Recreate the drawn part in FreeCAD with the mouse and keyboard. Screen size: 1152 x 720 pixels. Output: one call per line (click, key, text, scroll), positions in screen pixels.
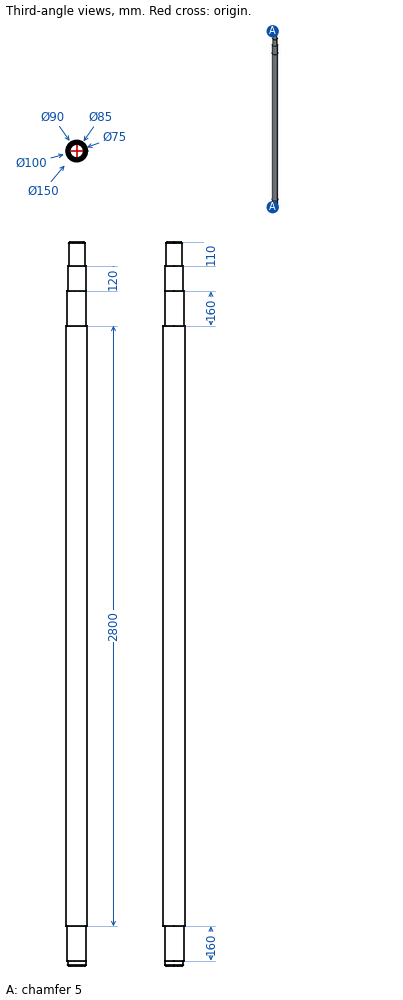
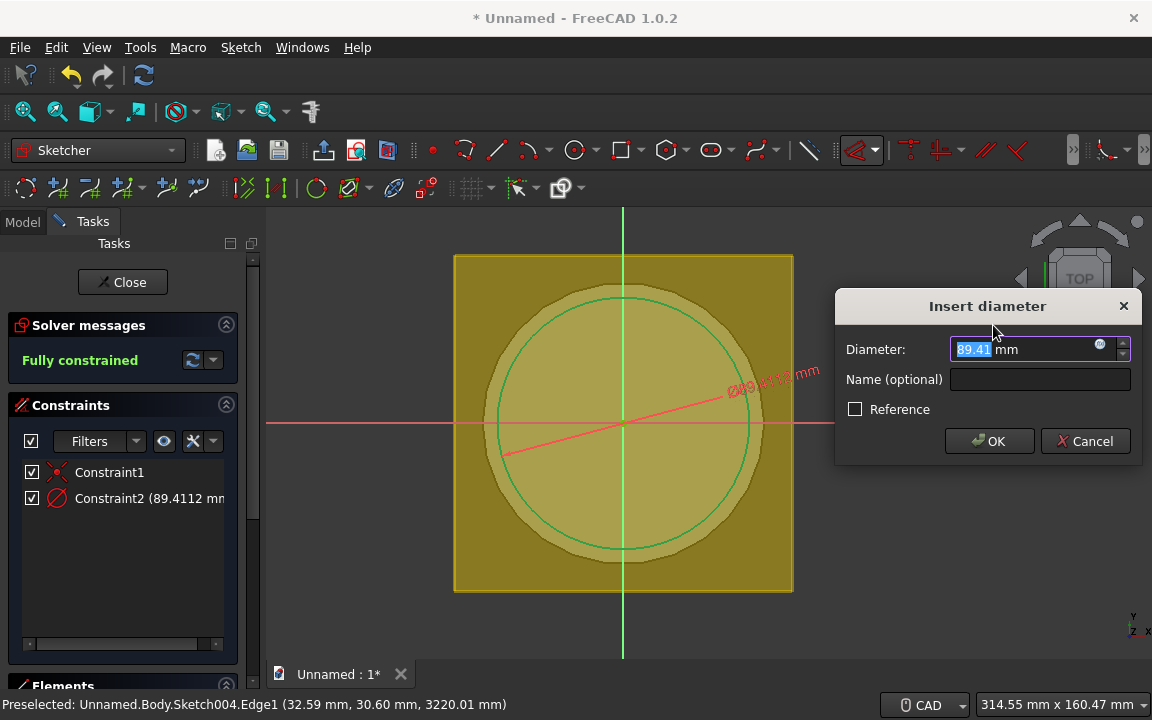
text(90)
key(Return)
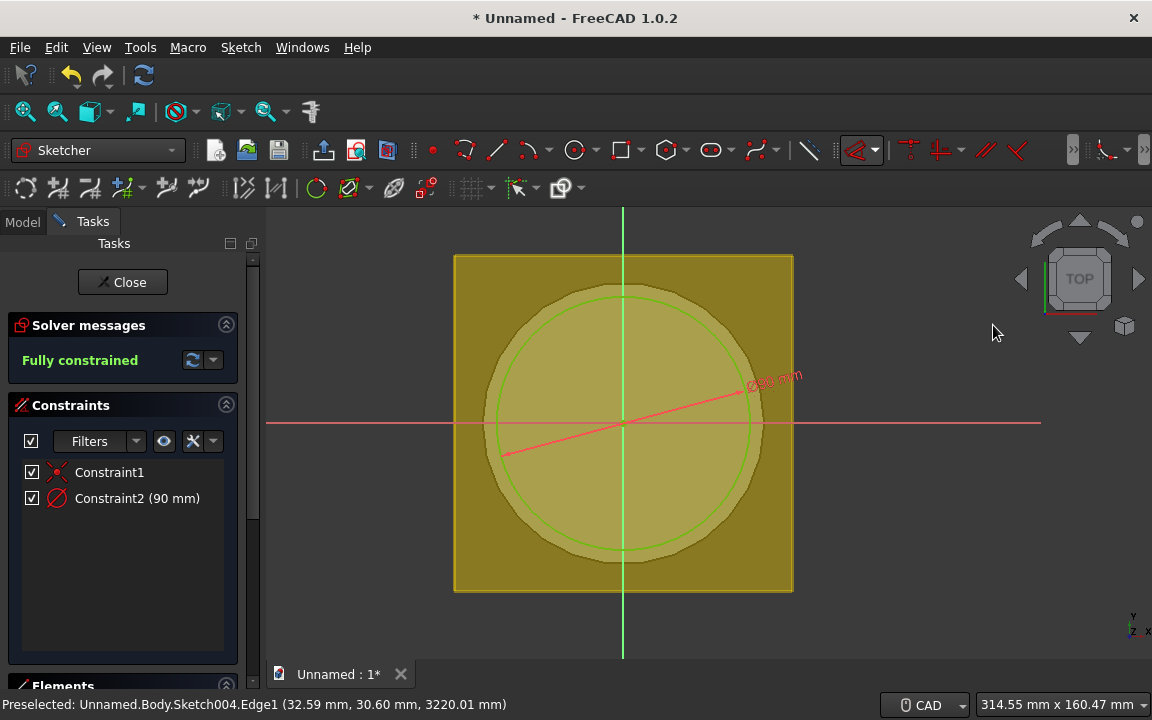
click(123, 282)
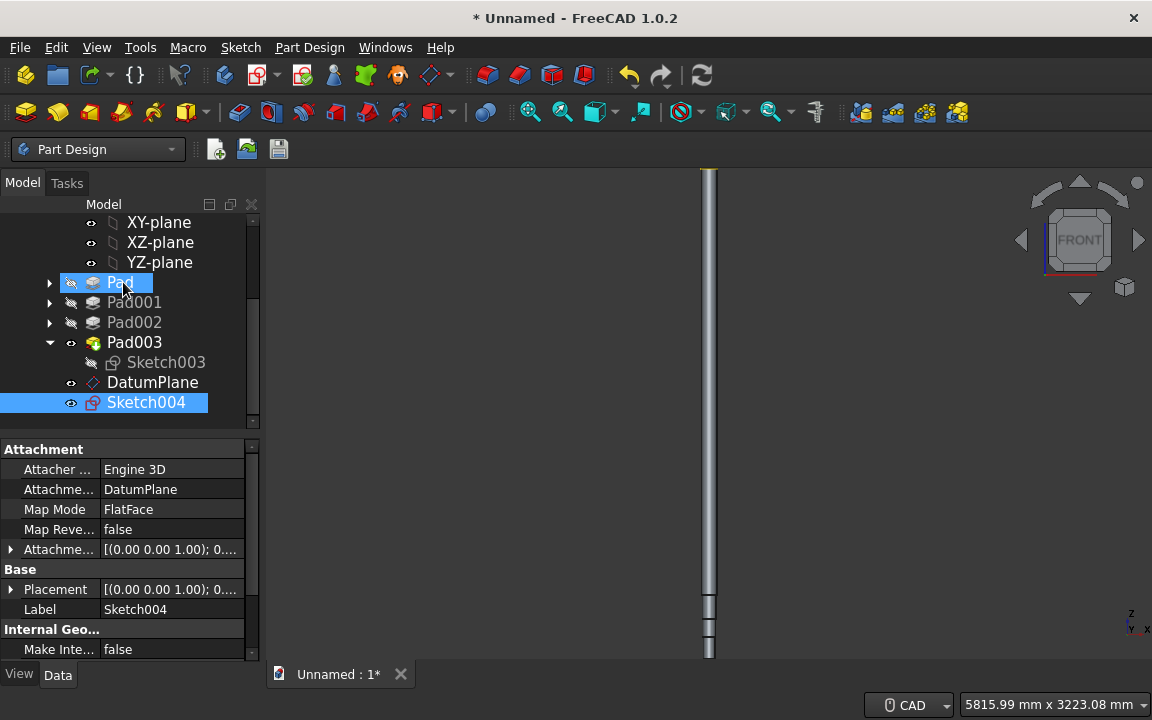
click(26, 112)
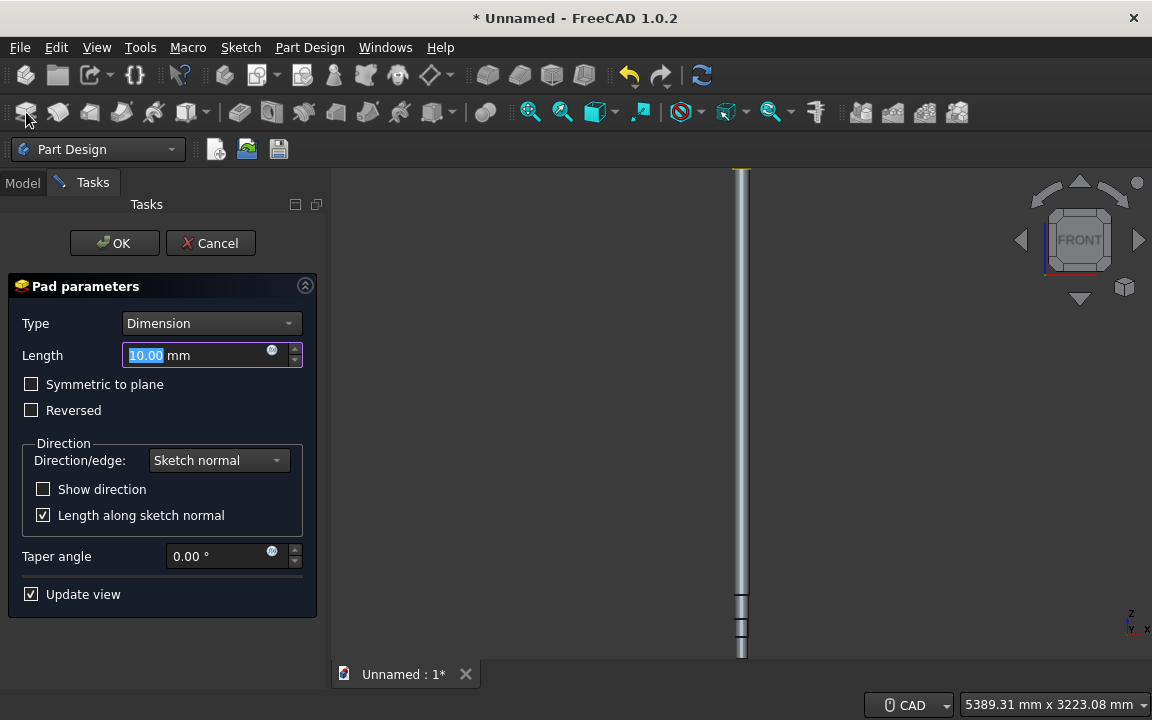
text(160)
key(Tab)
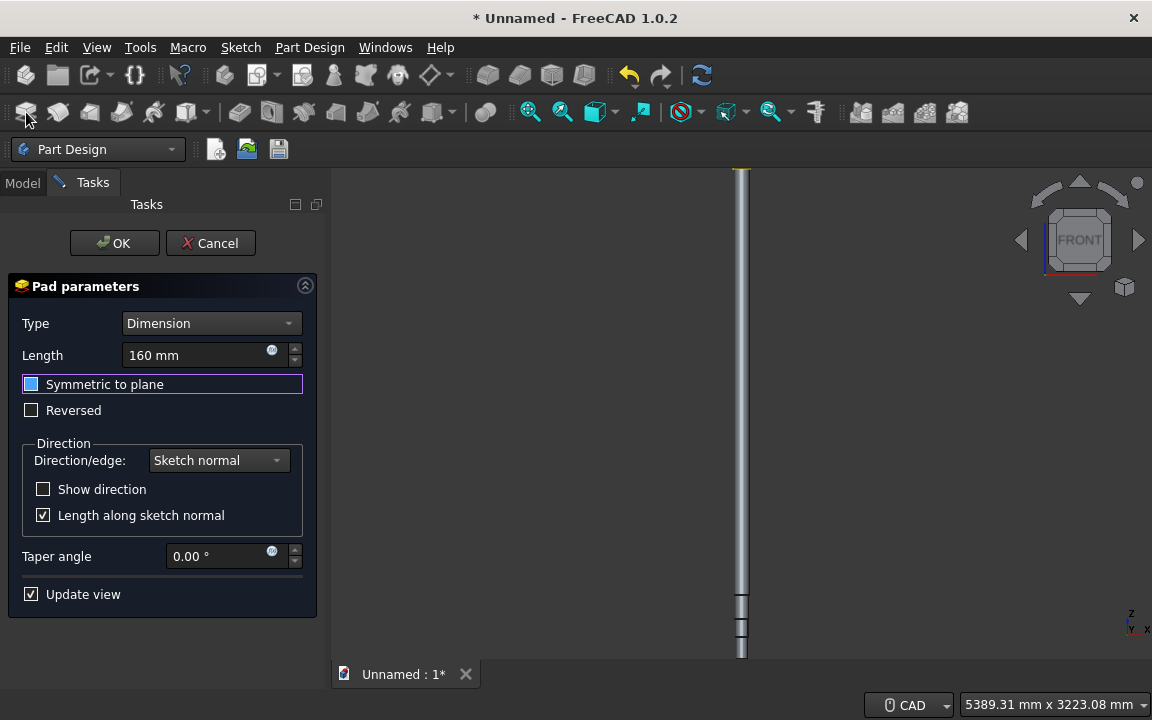
click(115, 243)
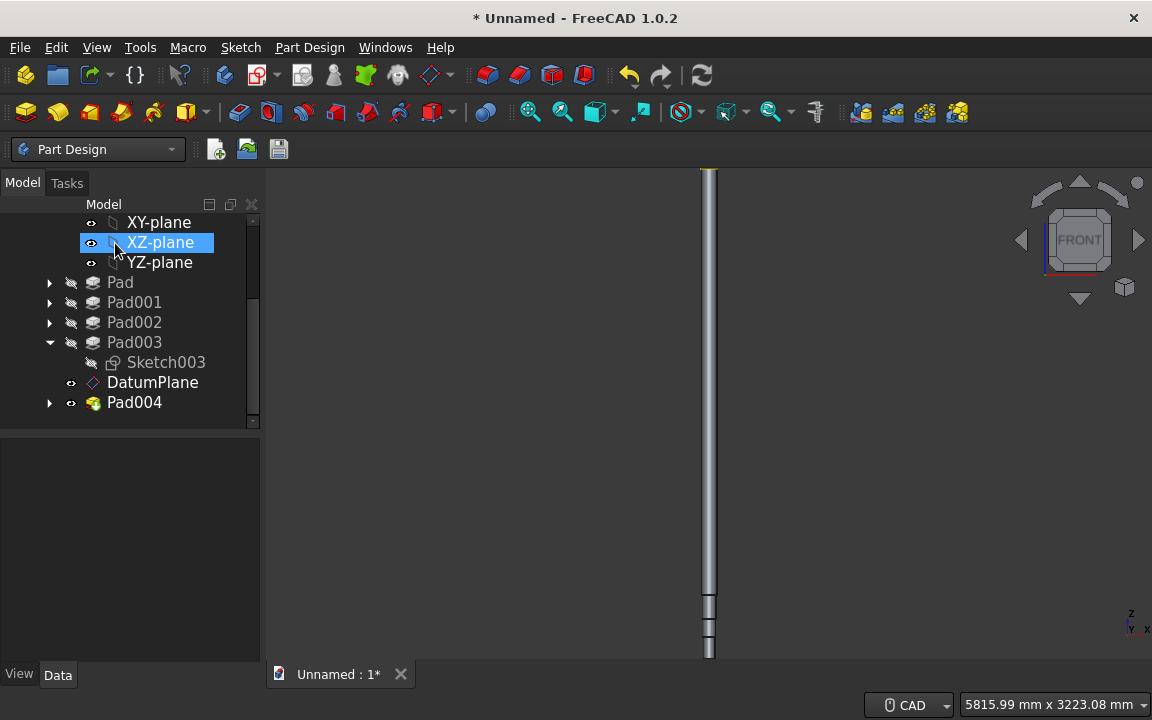
click(116, 383)
key(space)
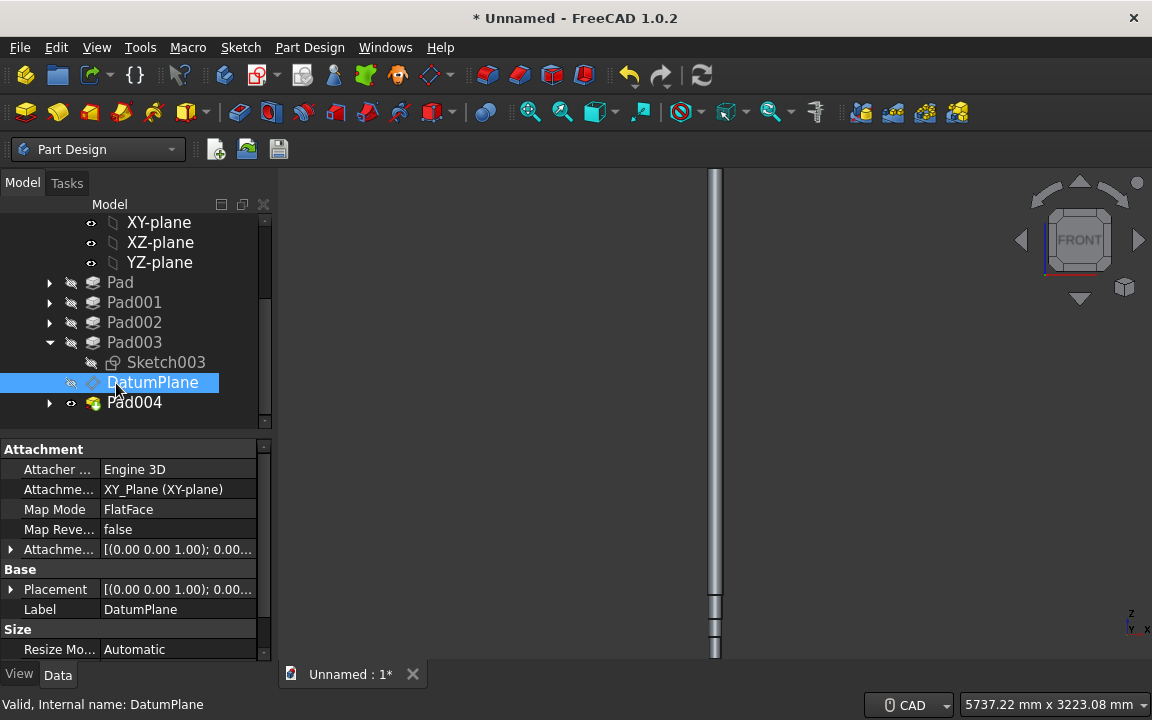
click(532, 112)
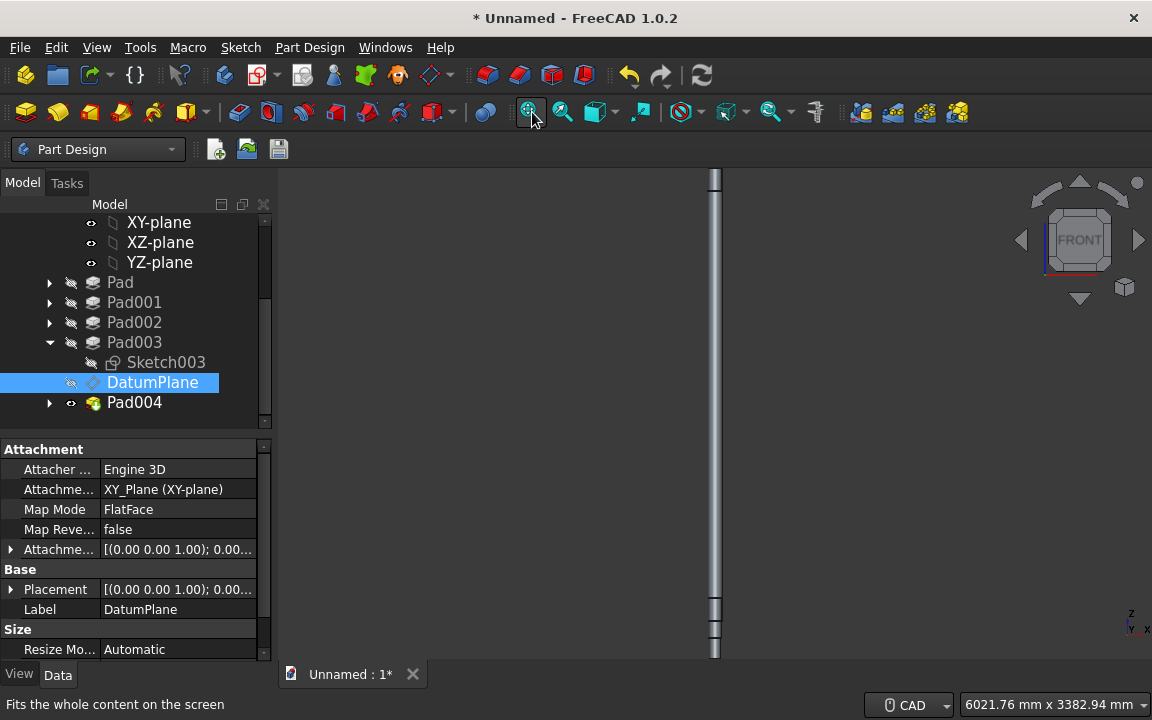
key(0)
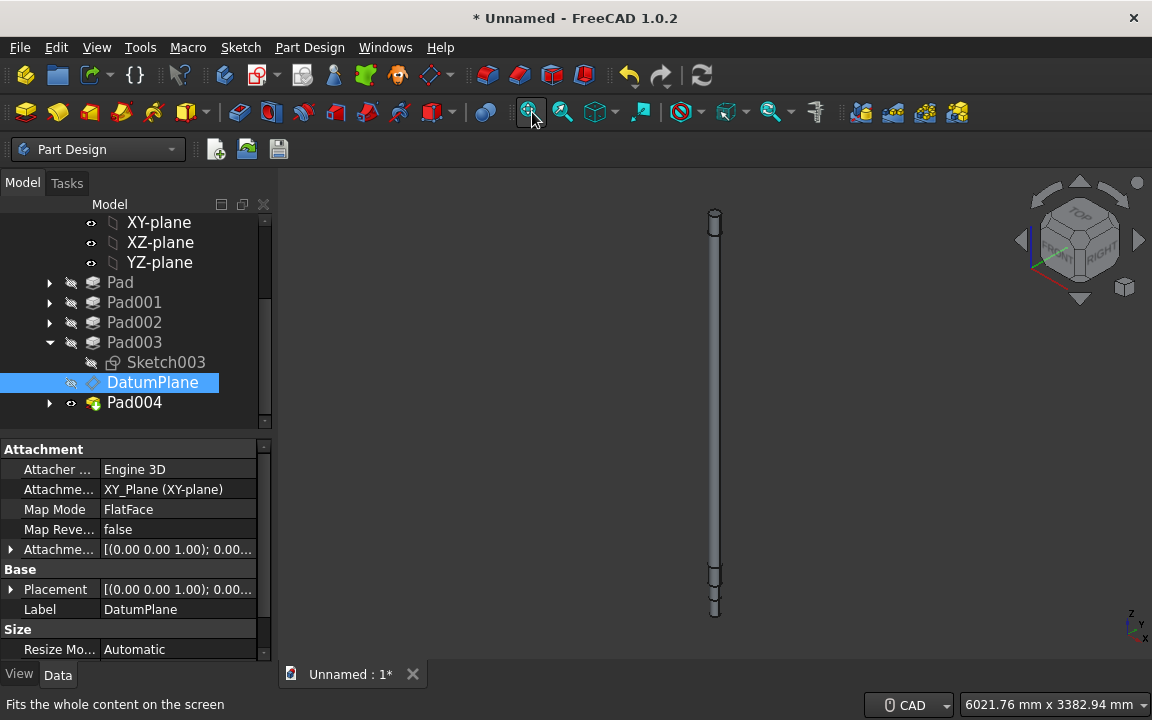
scroll(715, 212, up, 4)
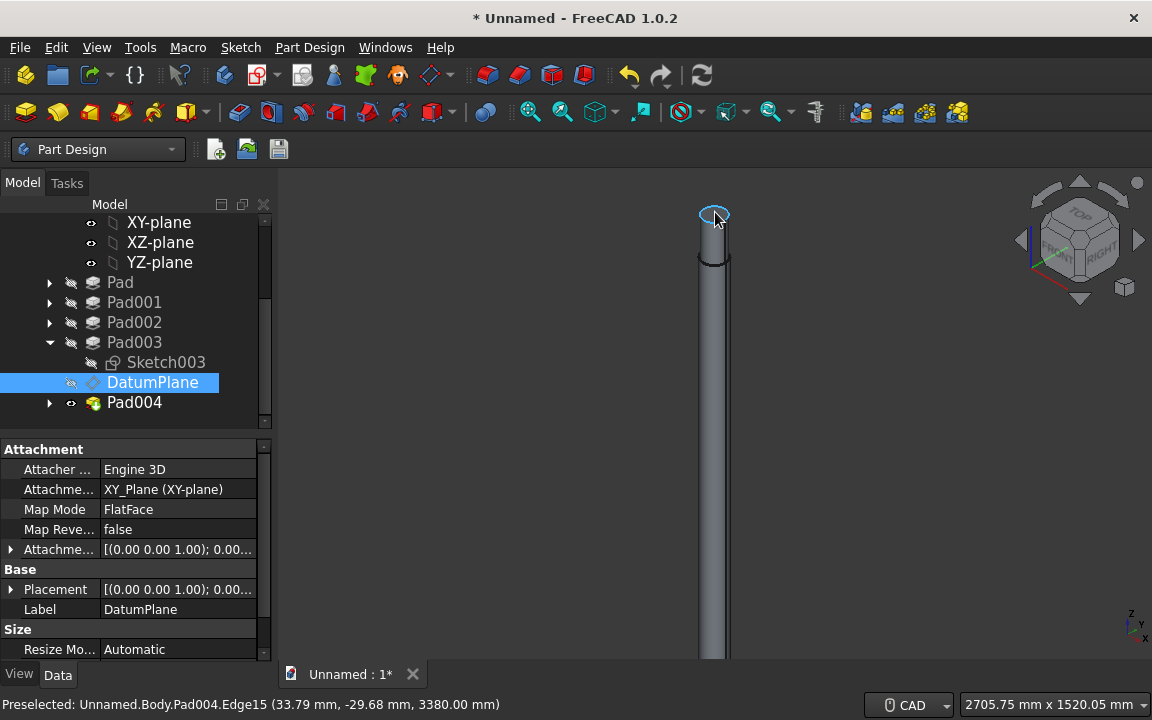
click(717, 212)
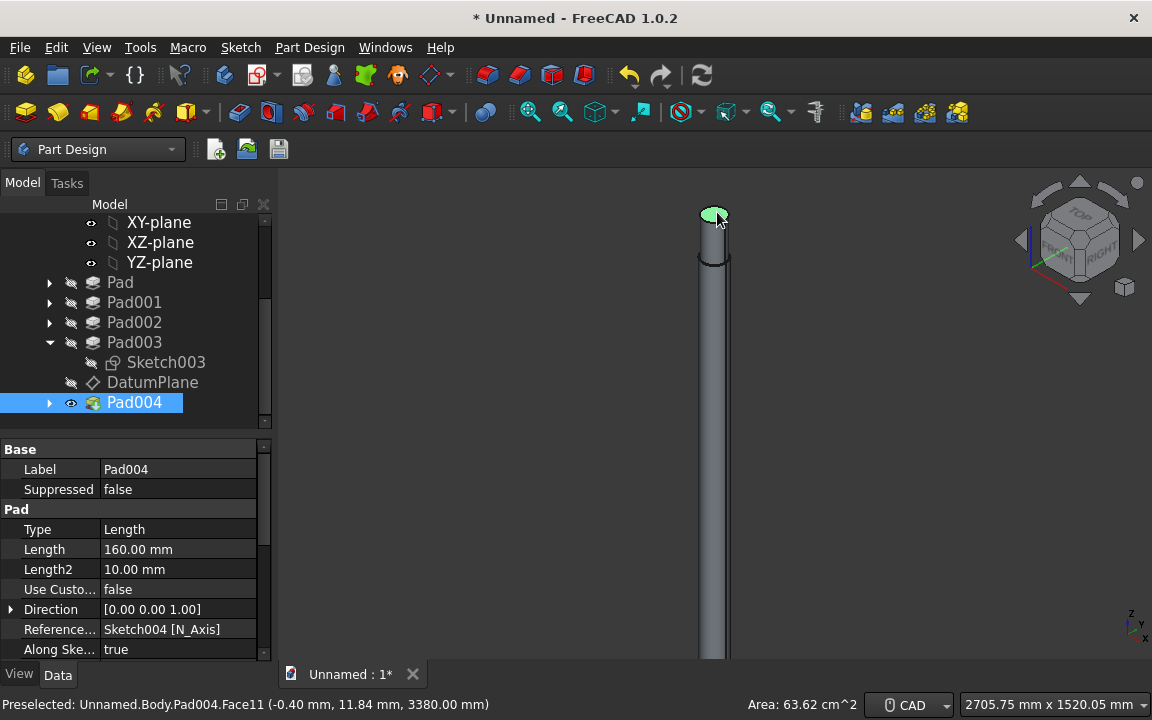
click(258, 76)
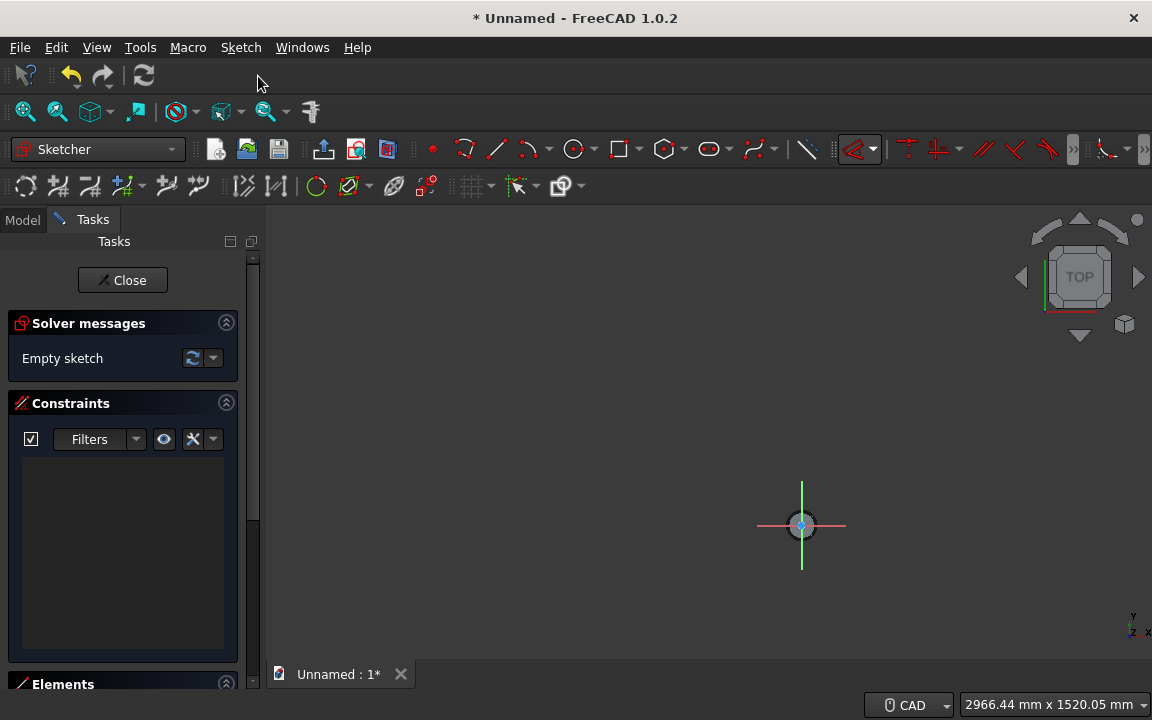
scroll(818, 535, up, 12)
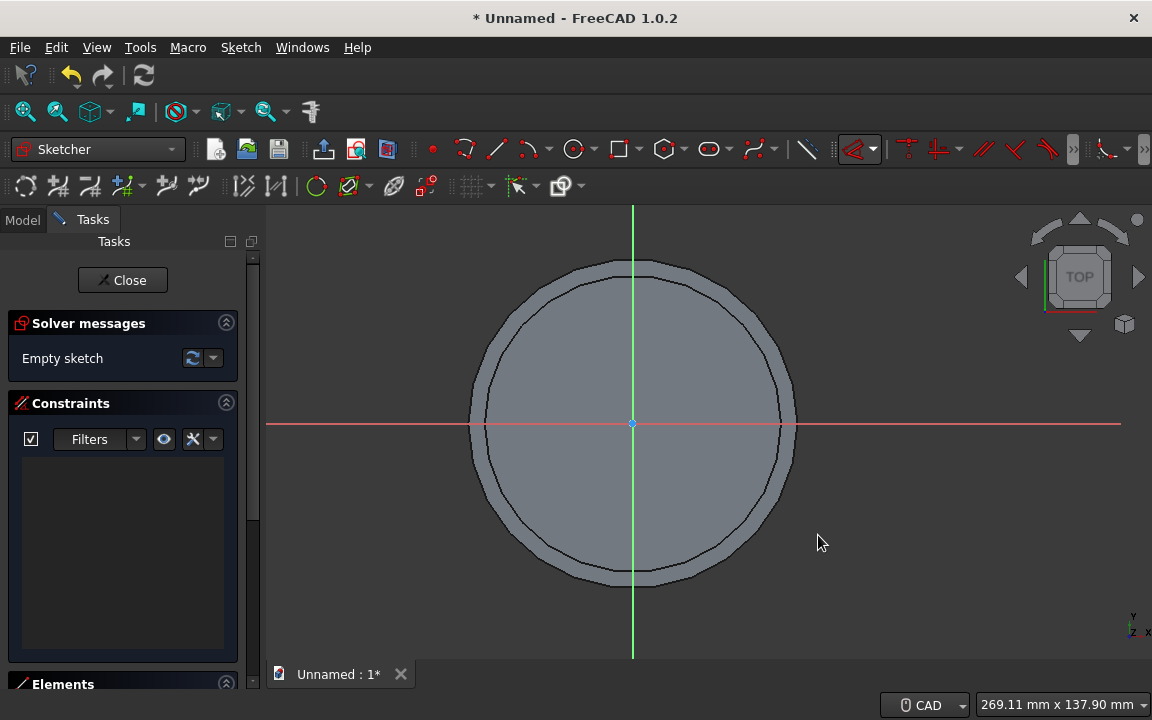
click(574, 150)